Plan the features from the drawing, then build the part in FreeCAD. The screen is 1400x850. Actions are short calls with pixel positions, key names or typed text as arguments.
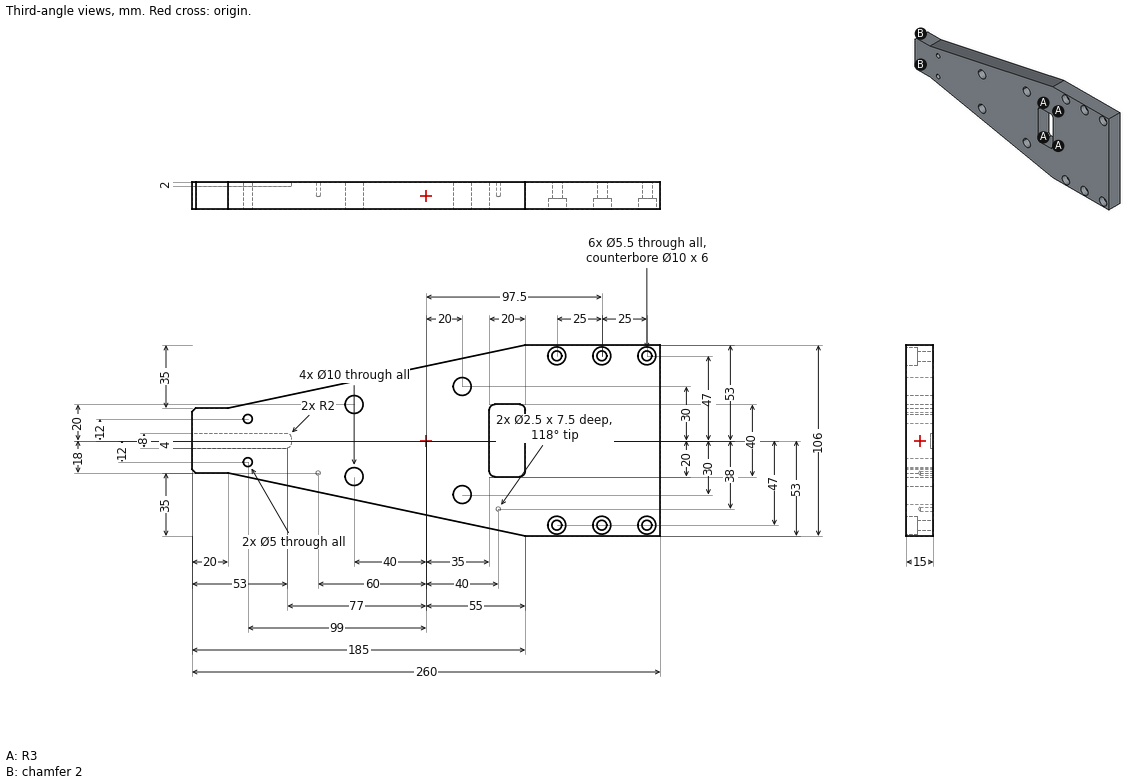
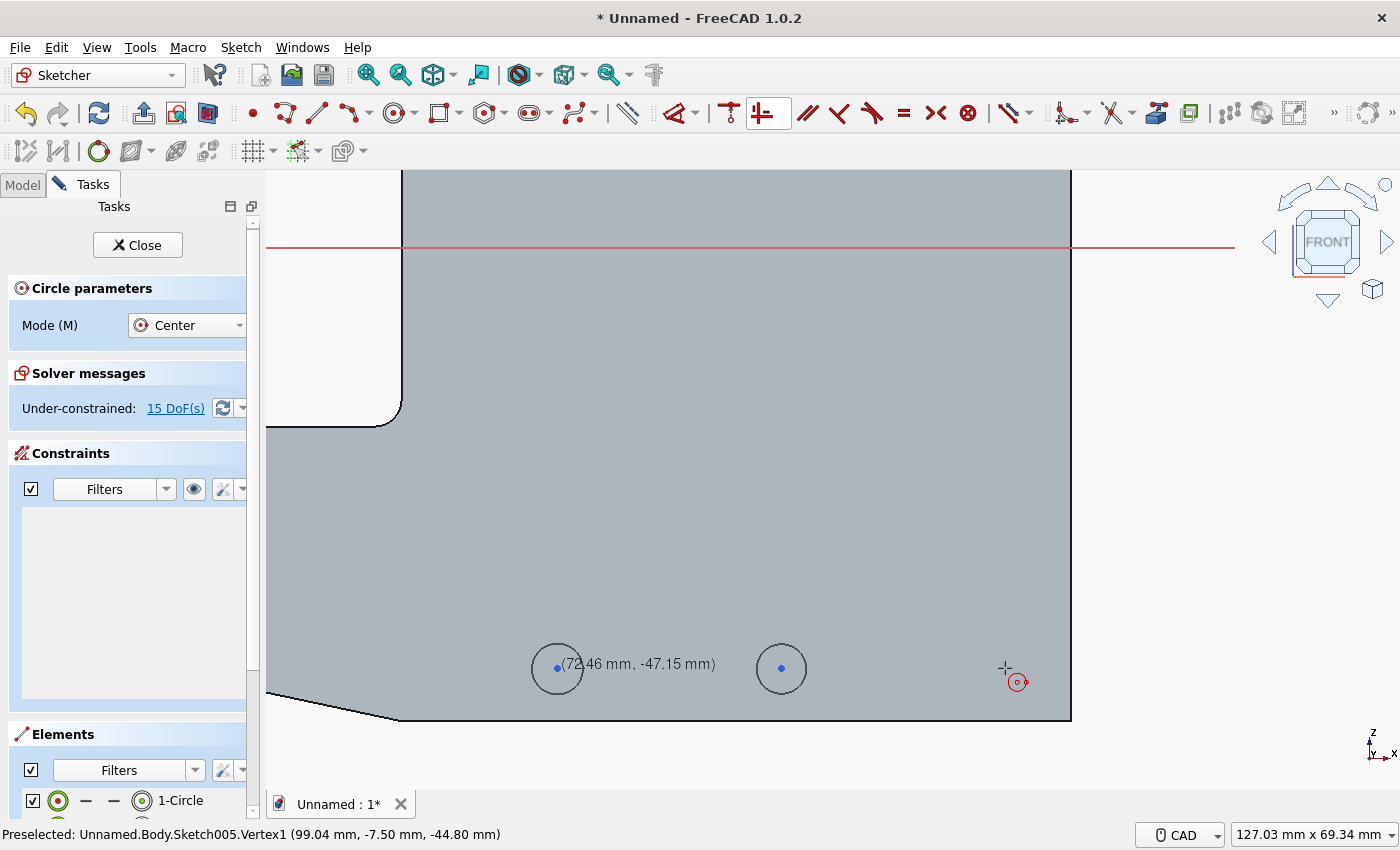
click(1004, 668)
click(1022, 650)
key(Escape)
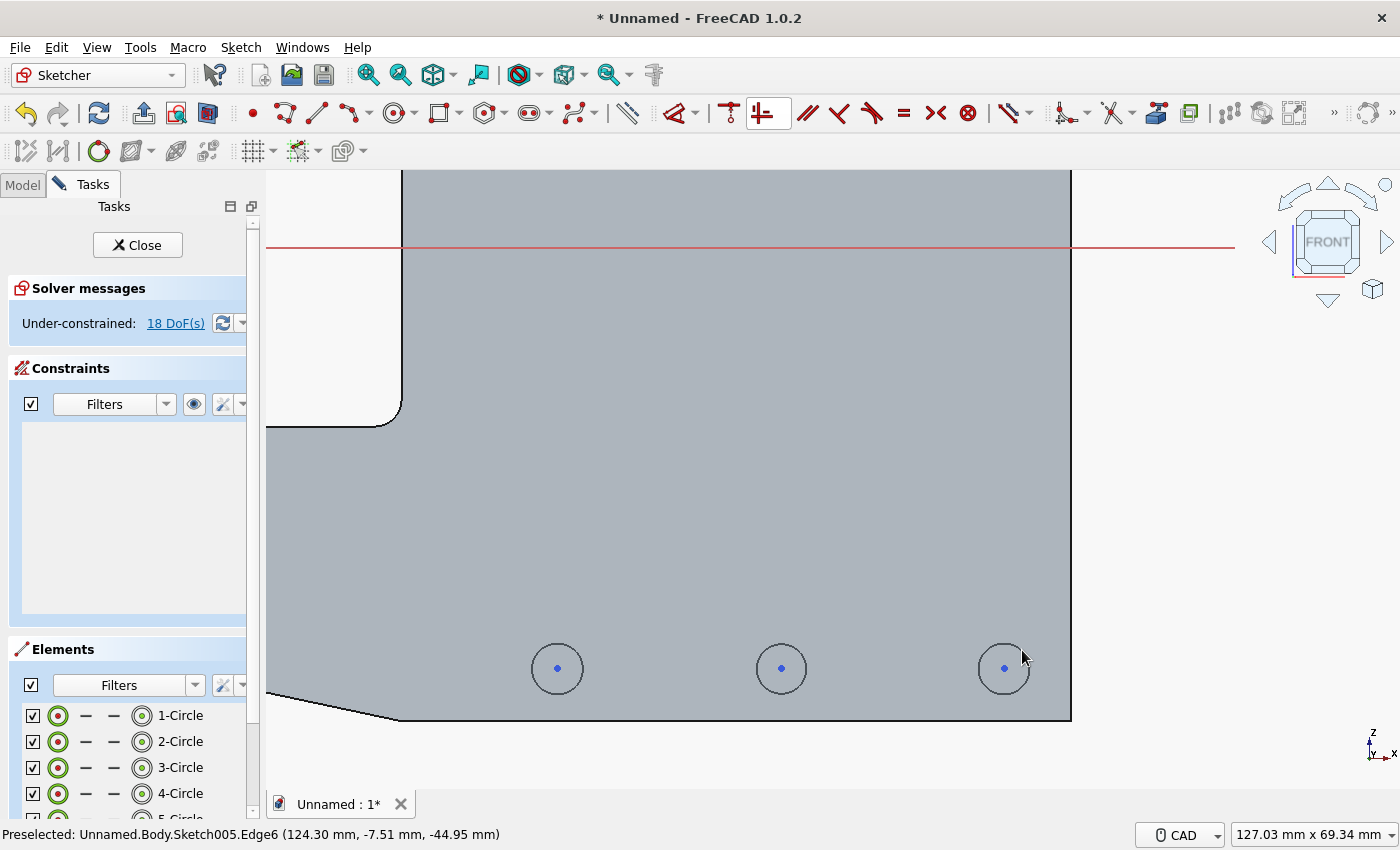
scroll(1005, 668, down, 4)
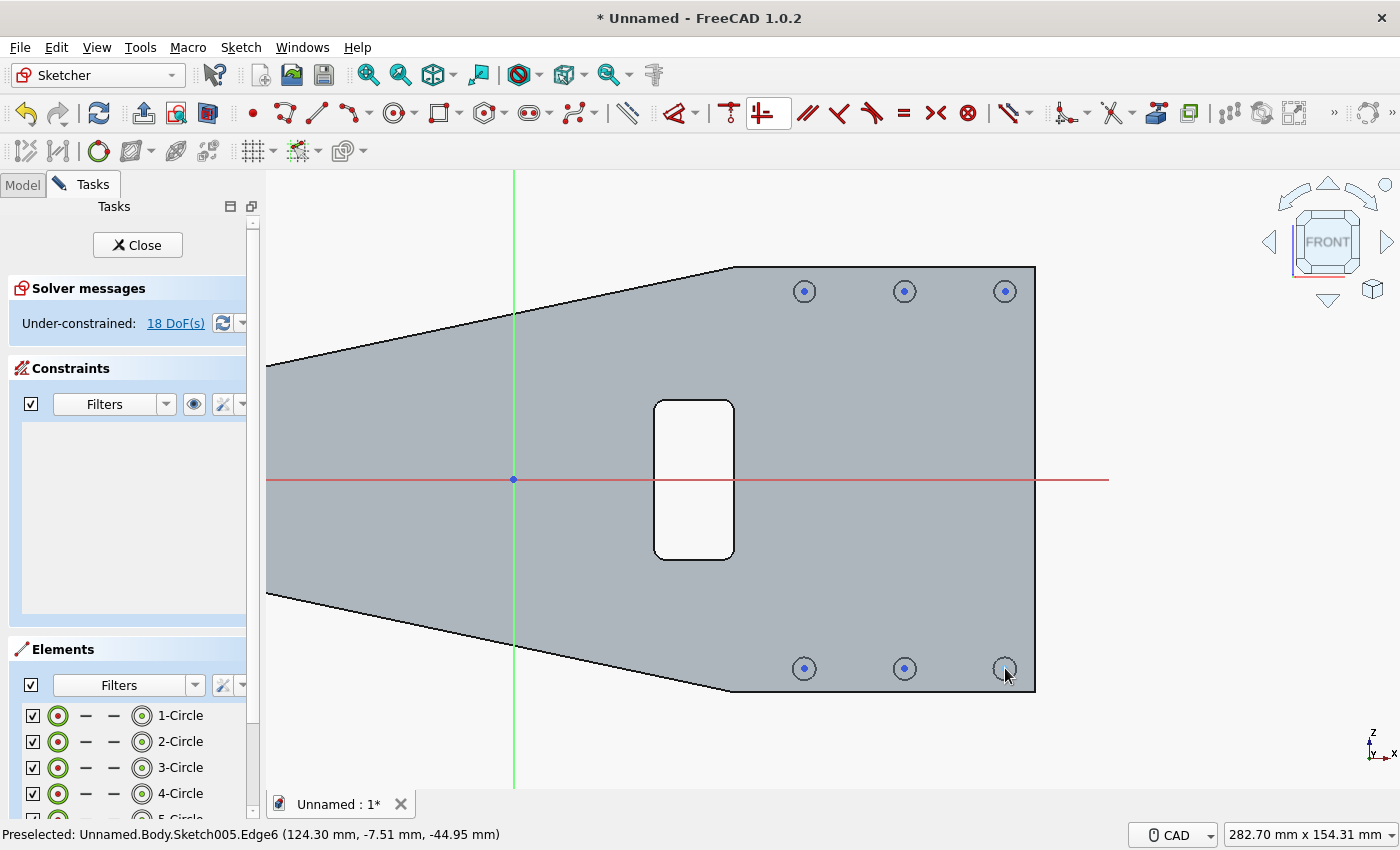
scroll(1013, 284, up, 2)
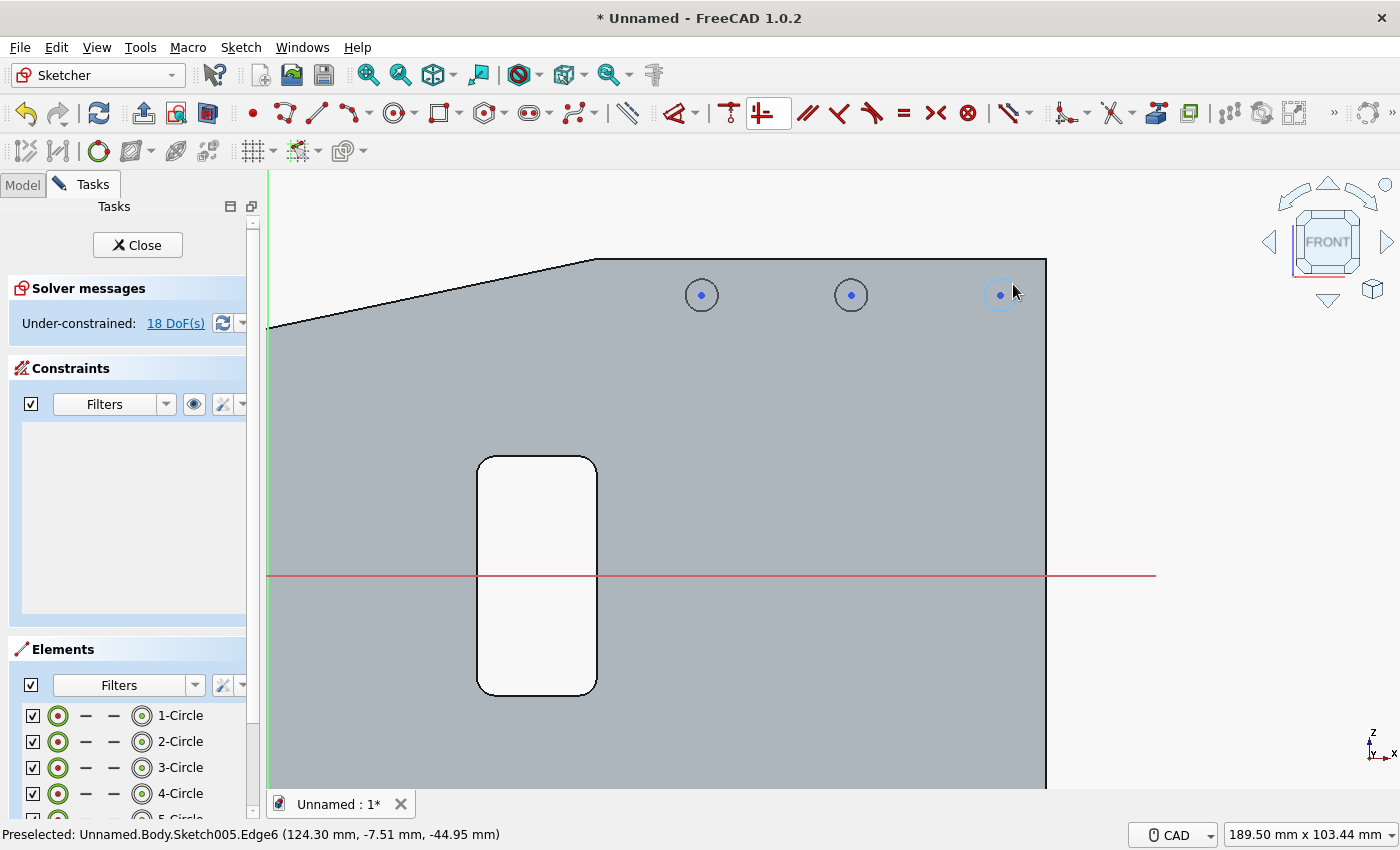
click(1012, 284)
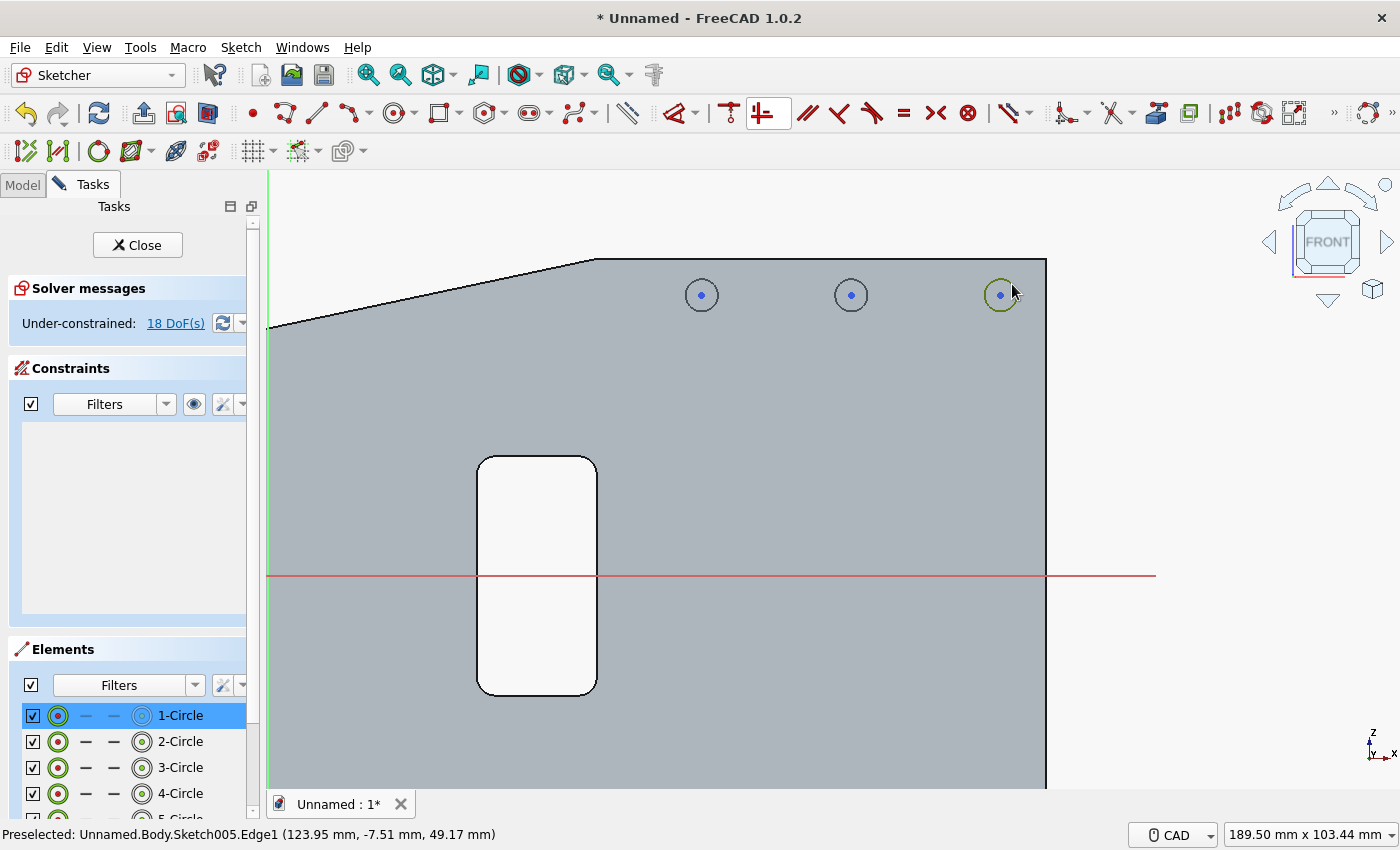
click(863, 284)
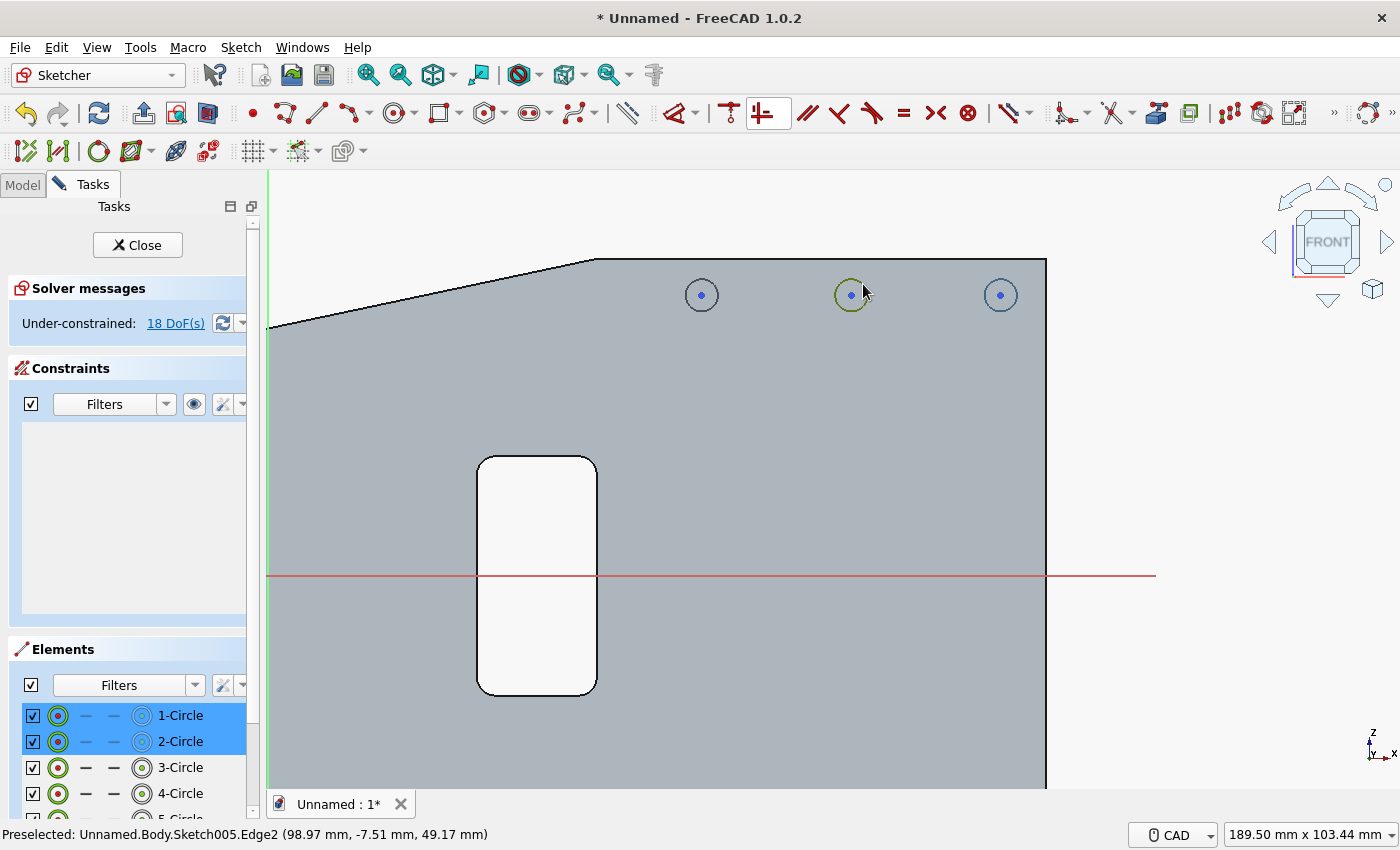
click(713, 284)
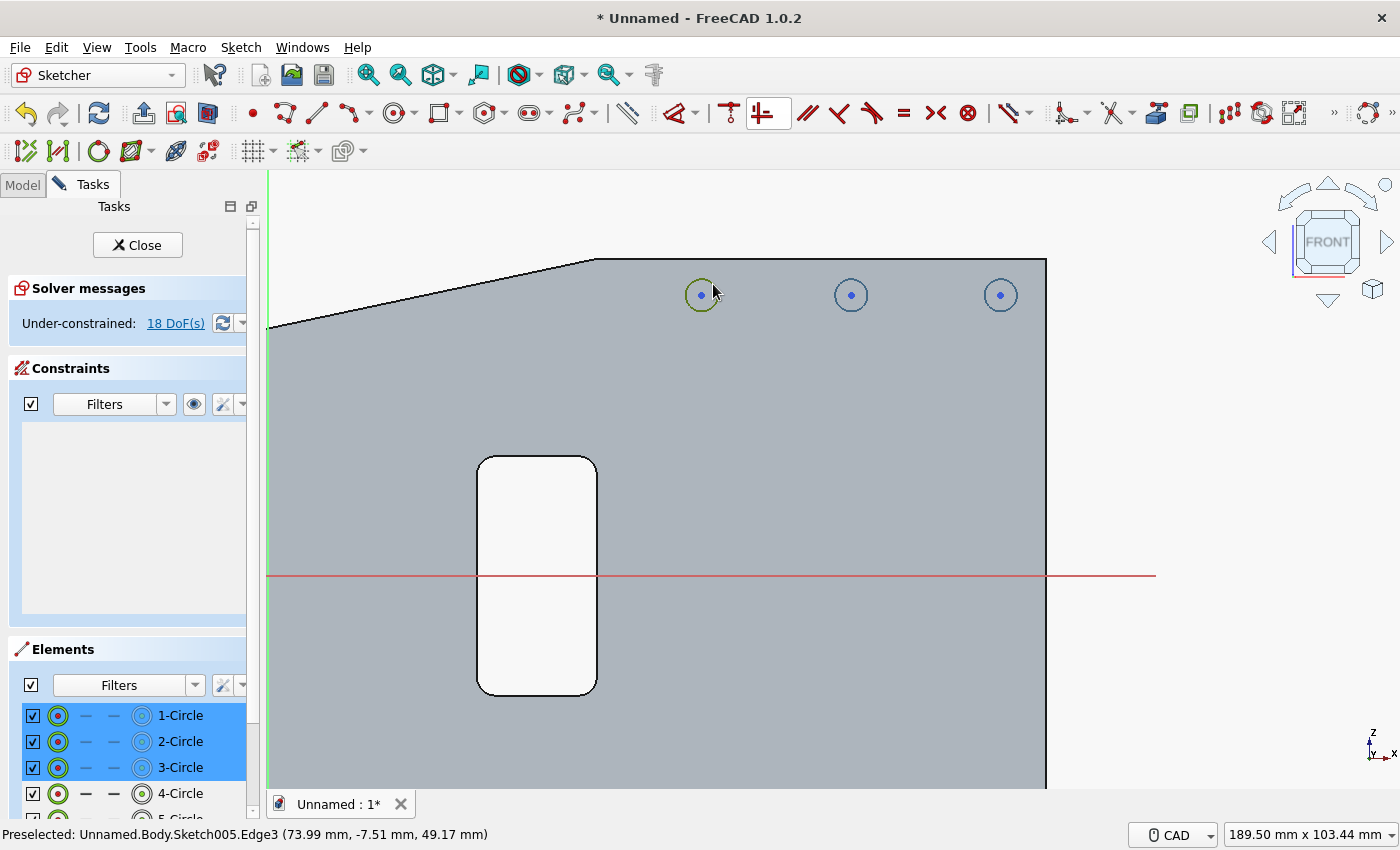
scroll(1013, 283, down, 2)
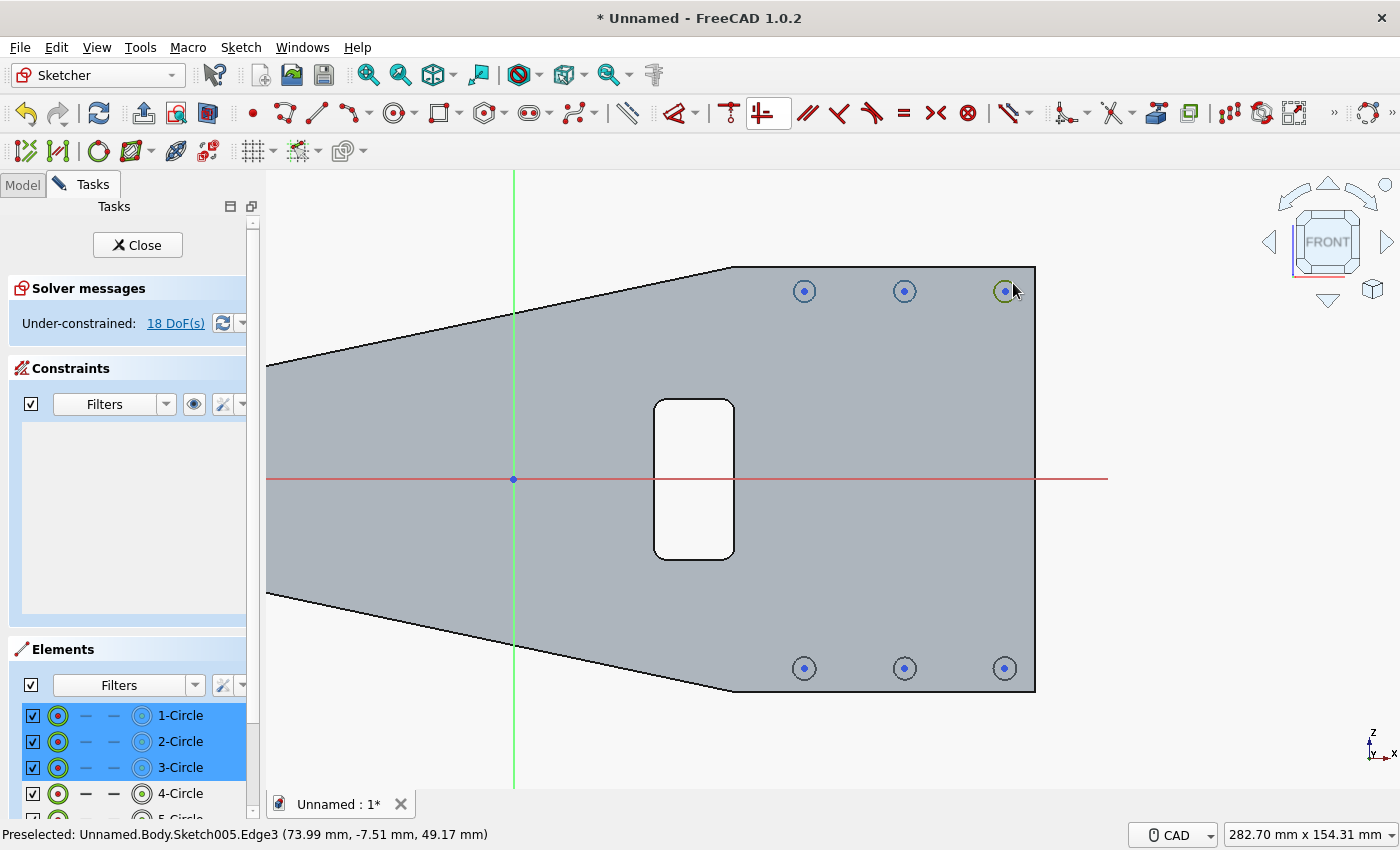
click(812, 660)